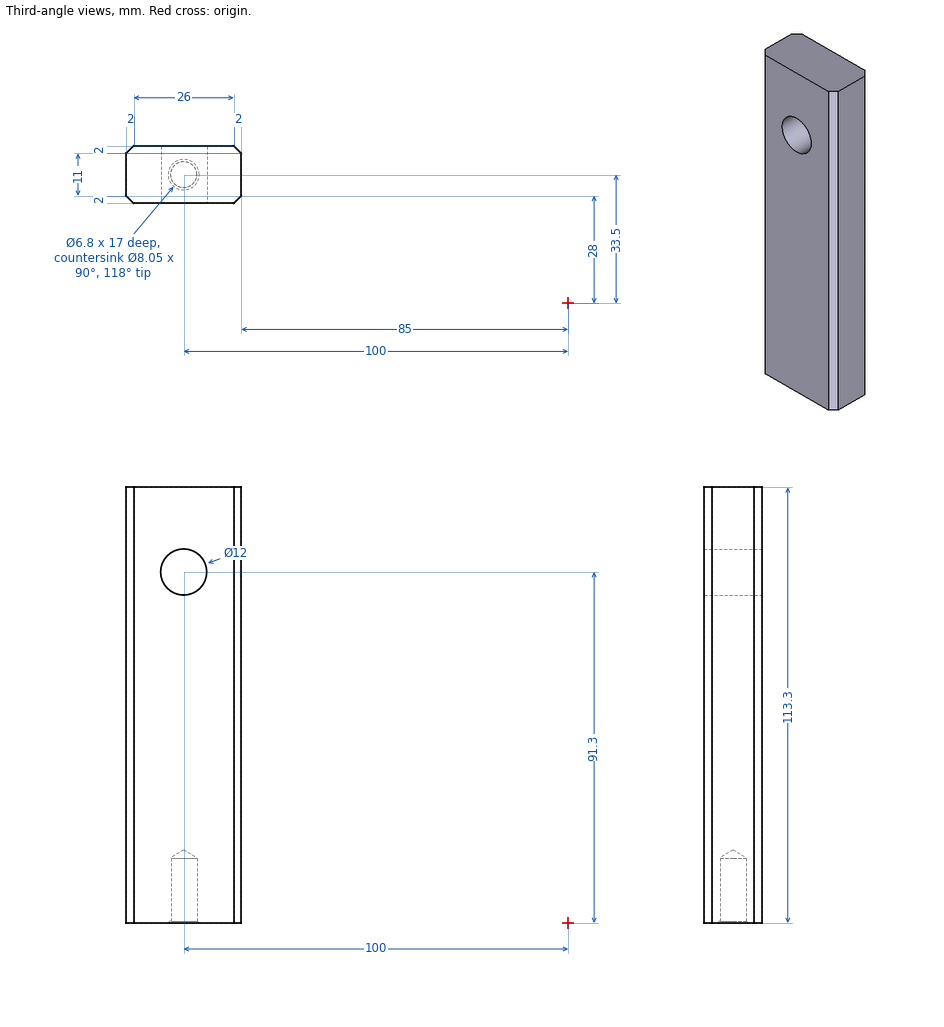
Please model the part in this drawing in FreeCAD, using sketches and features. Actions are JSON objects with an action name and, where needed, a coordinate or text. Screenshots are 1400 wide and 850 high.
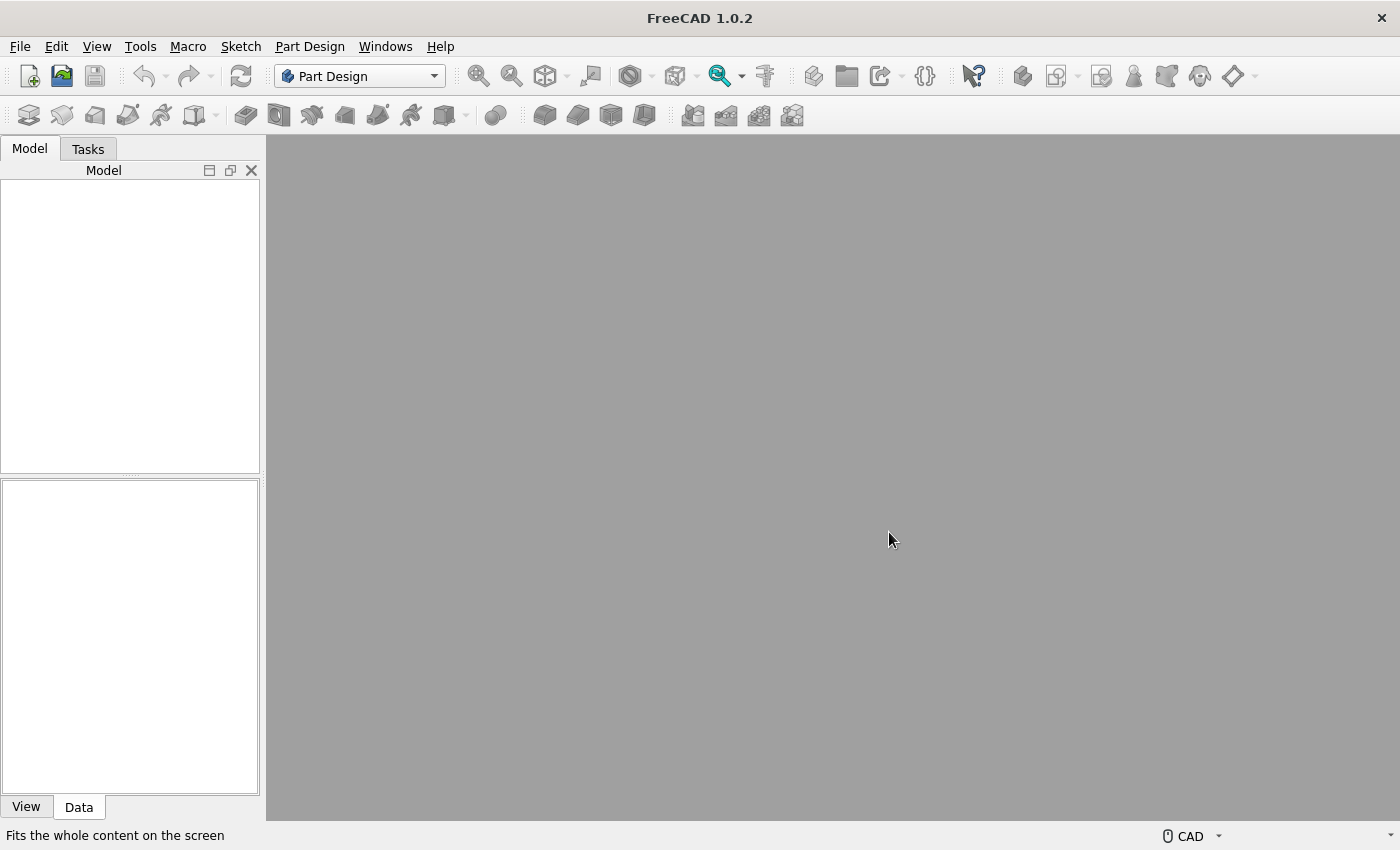
{"action": "left_click", "coordinate": [29, 76]}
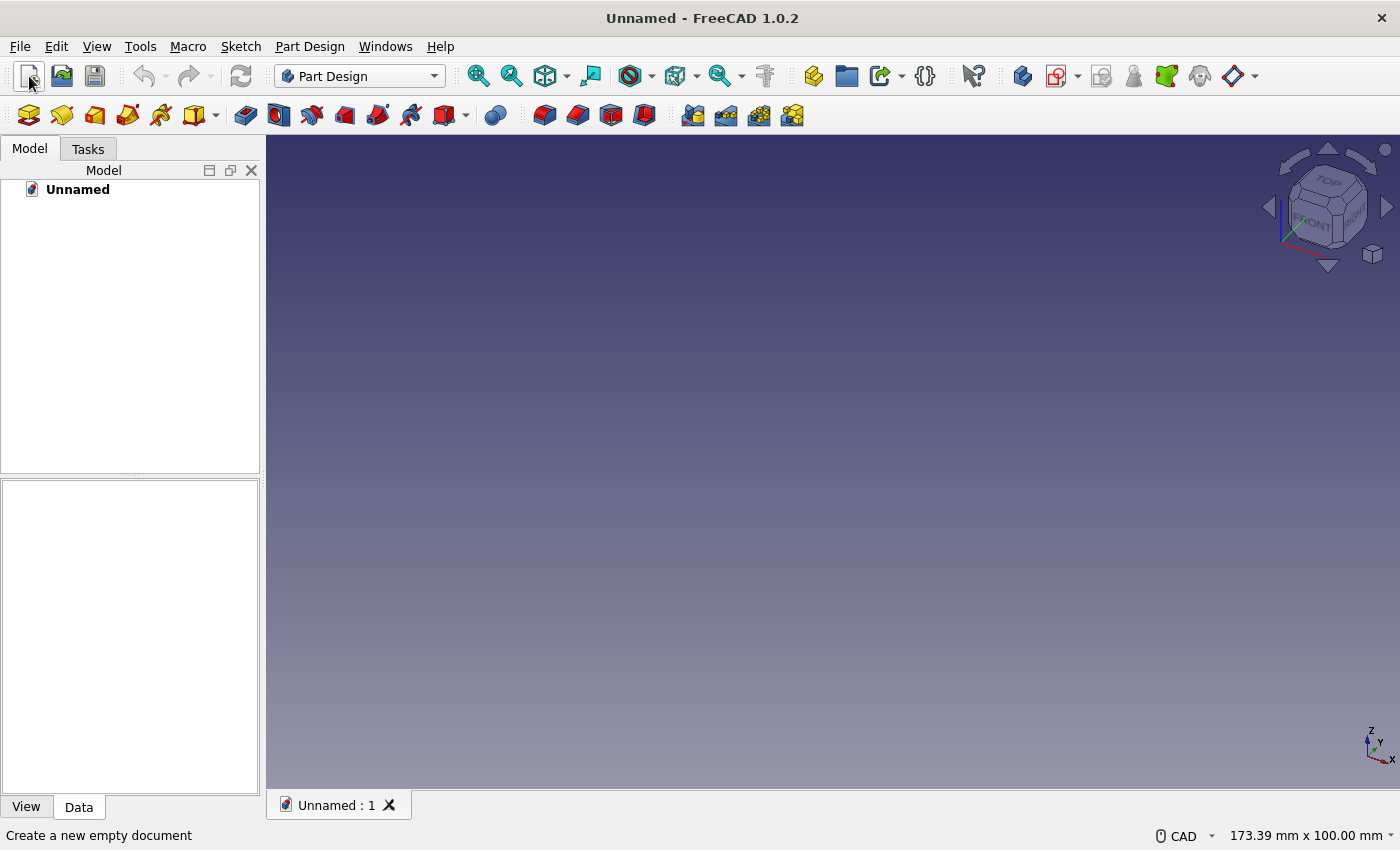
{"action": "left_click", "coordinate": [1056, 76]}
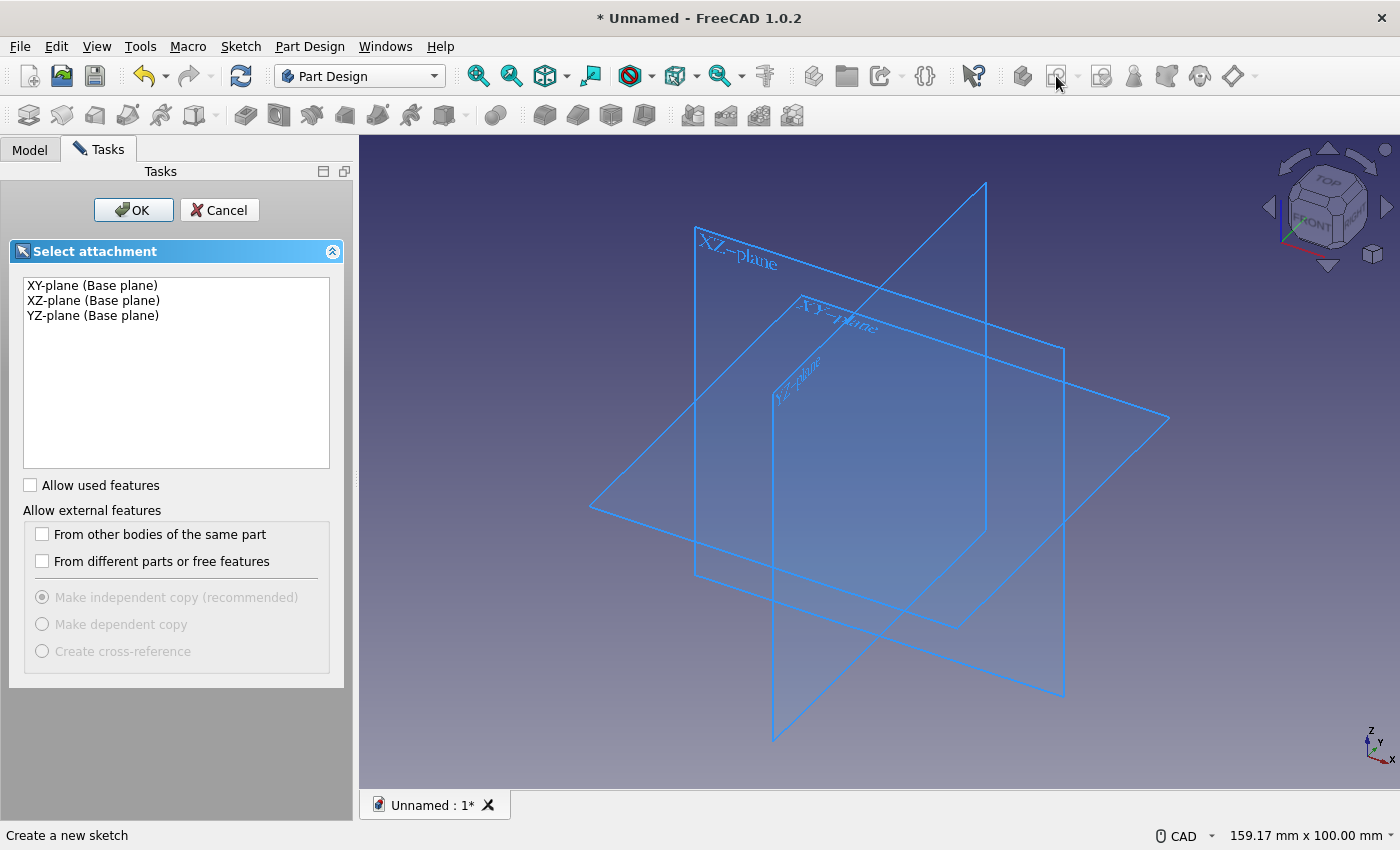
{"action": "left_click", "coordinate": [84, 286]}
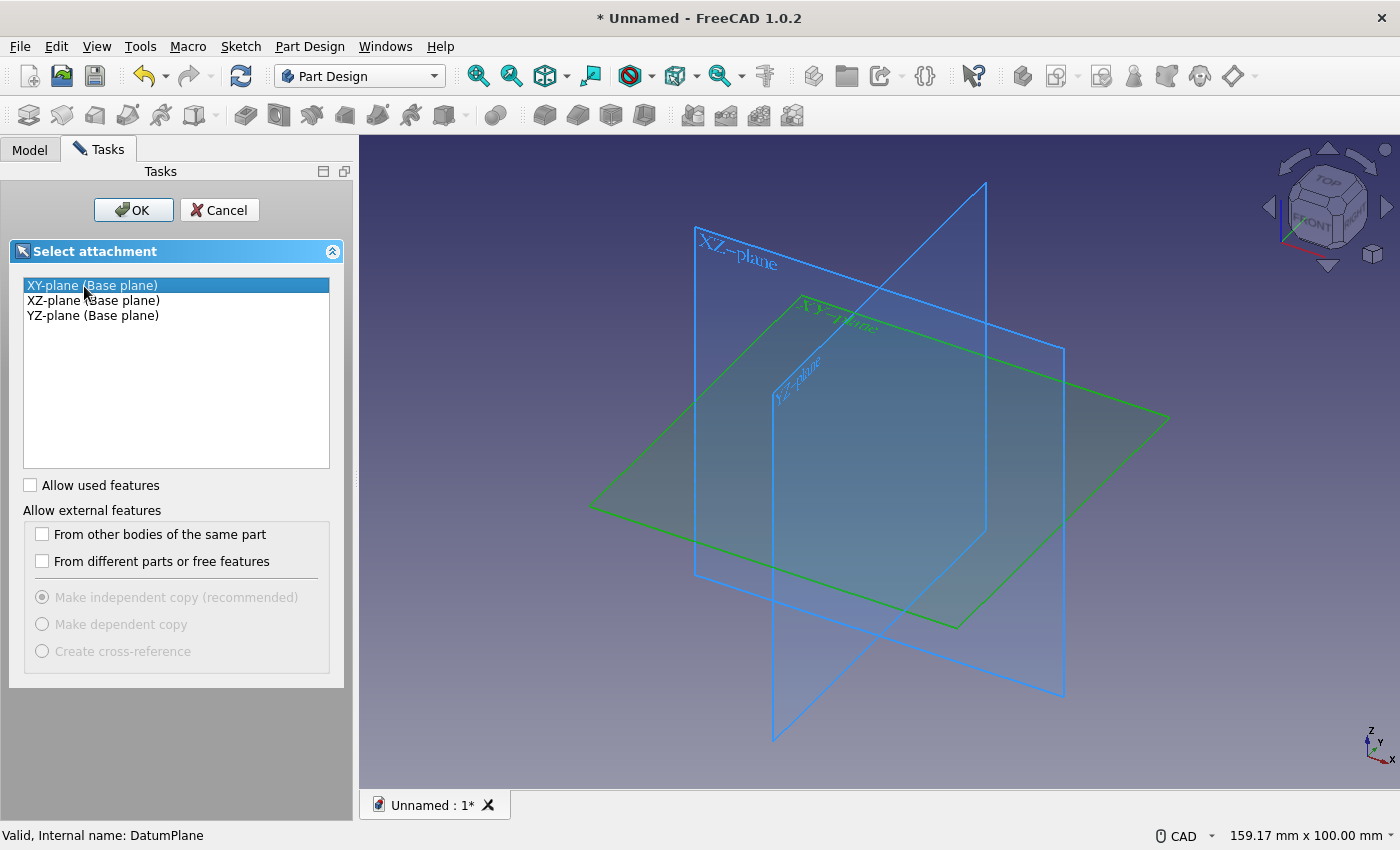
{"action": "left_click", "coordinate": [134, 210]}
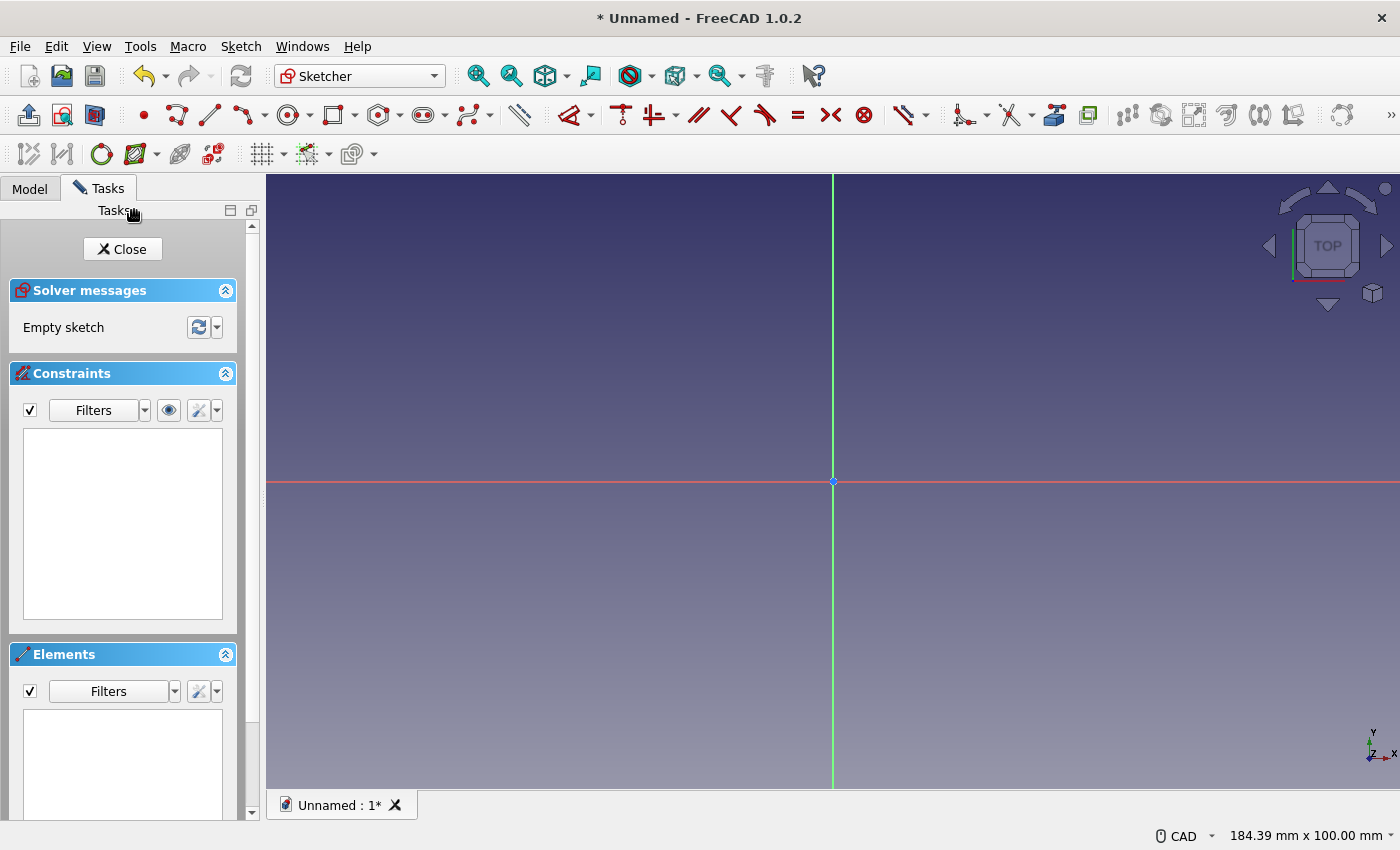
{"action": "scroll", "coordinate": [764, 482], "scroll_direction": "down", "scroll_amount": 5}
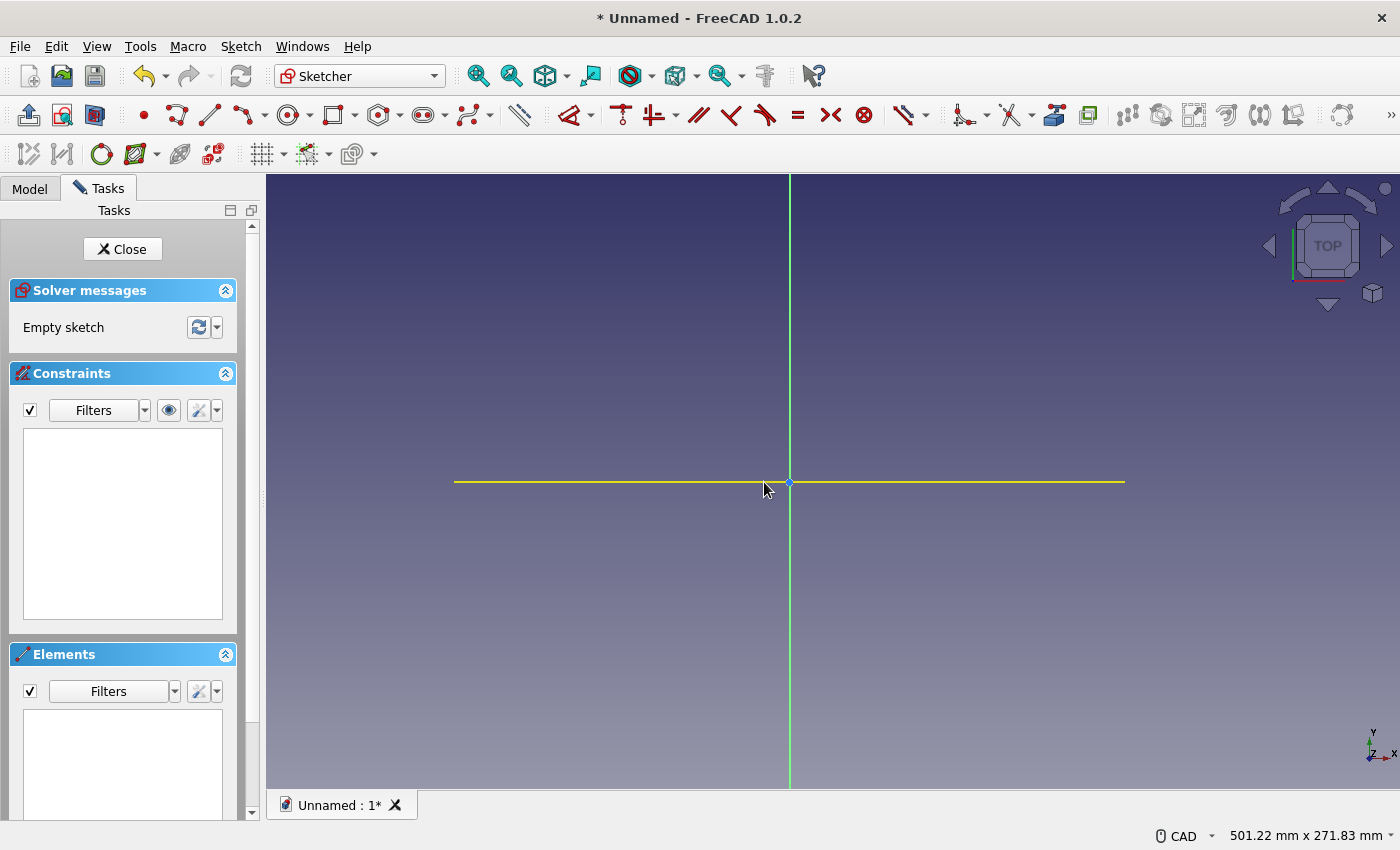
{"action": "scroll", "coordinate": [538, 397], "scroll_direction": "up", "scroll_amount": 11}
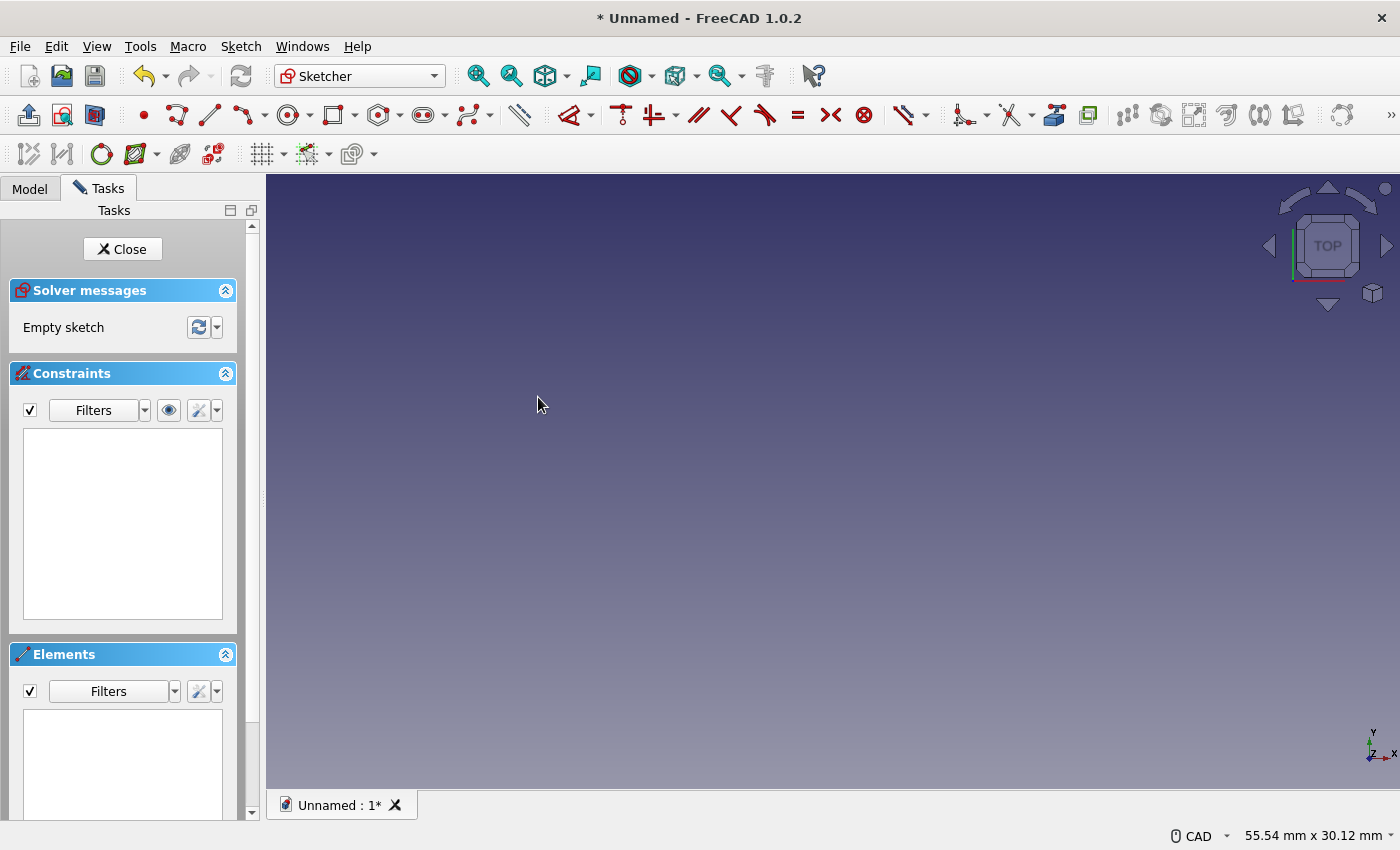
{"action": "left_click", "coordinate": [177, 116]}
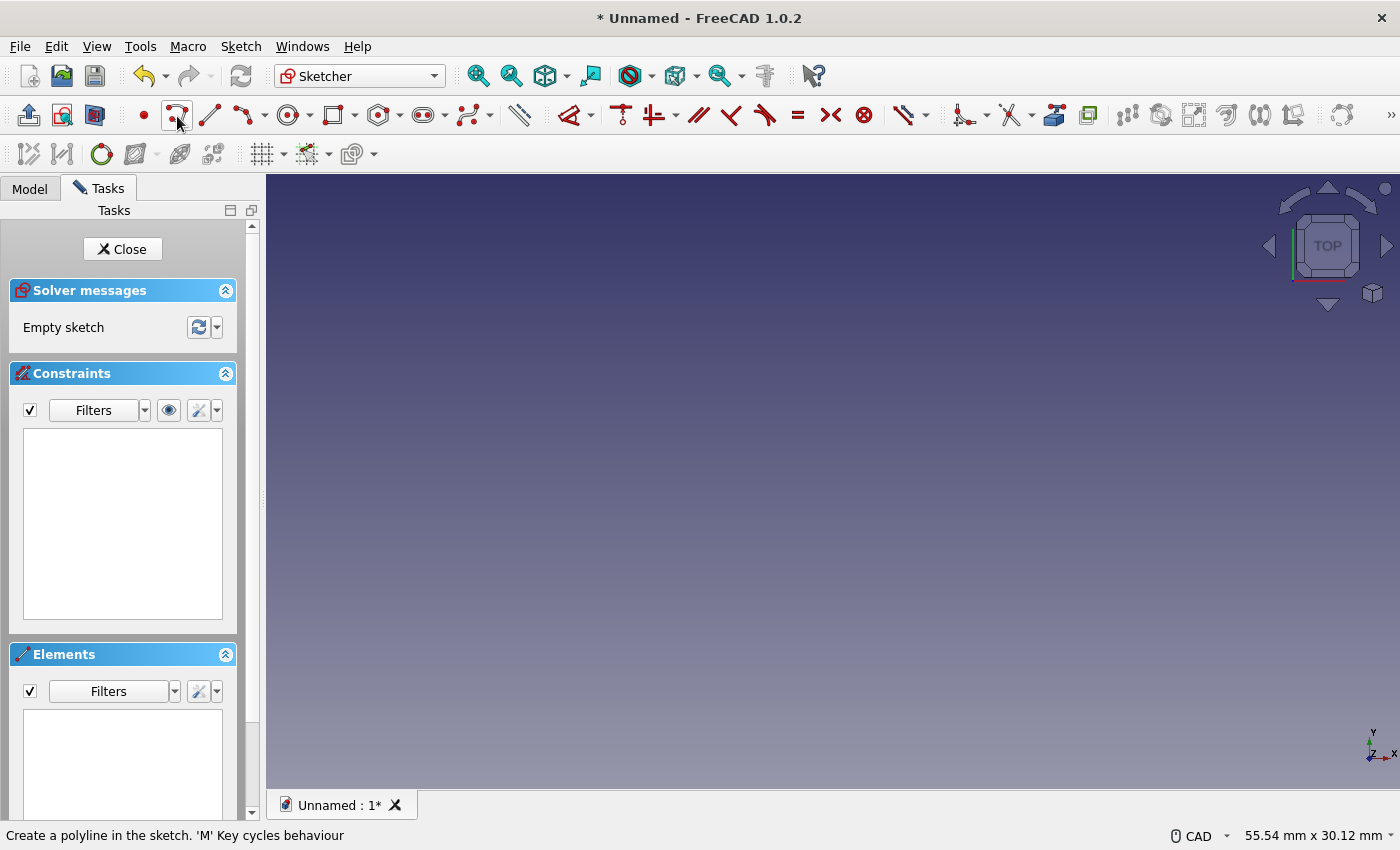
{"action": "left_click", "coordinate": [1072, 591]}
{"action": "left_click", "coordinate": [1072, 366]}
{"action": "left_click", "coordinate": [1031, 325]}
{"action": "left_click", "coordinate": [500, 325]}
{"action": "left_click", "coordinate": [459, 366]}
{"action": "left_click", "coordinate": [459, 591]}
{"action": "left_click", "coordinate": [500, 632]}
{"action": "left_click", "coordinate": [1031, 632]}
{"action": "left_click", "coordinate": [1072, 592]}
{"action": "key", "text": "Escape"}
{"action": "key", "text": "Escape"}